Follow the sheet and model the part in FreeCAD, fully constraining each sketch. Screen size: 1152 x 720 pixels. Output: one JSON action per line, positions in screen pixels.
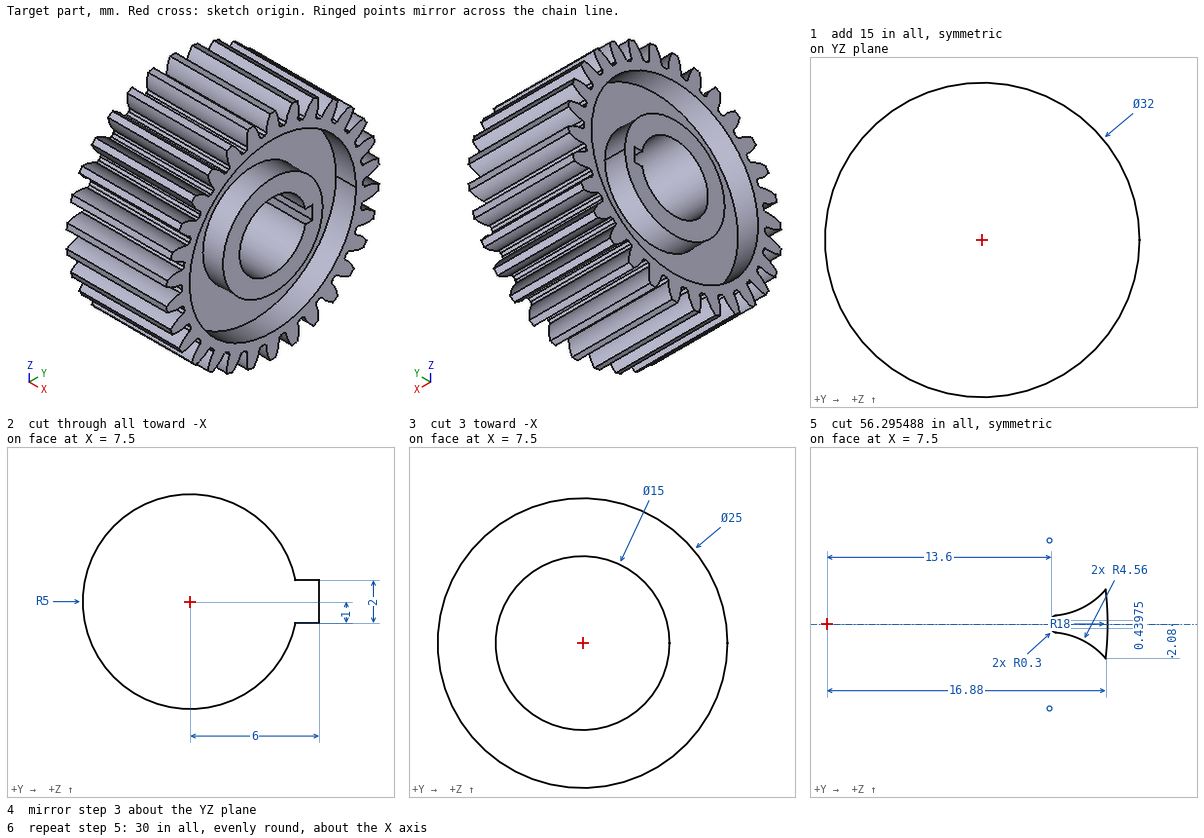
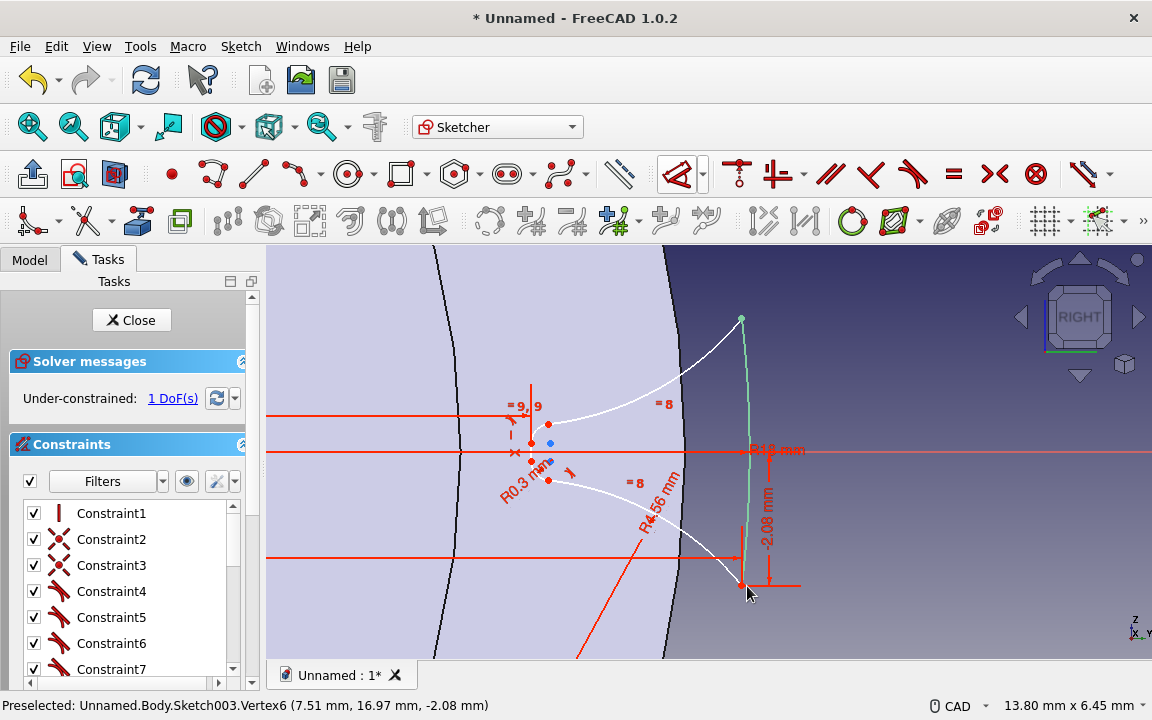
{"action": "scroll", "coordinate": [531, 452], "scroll_direction": "up", "scroll_amount": 3}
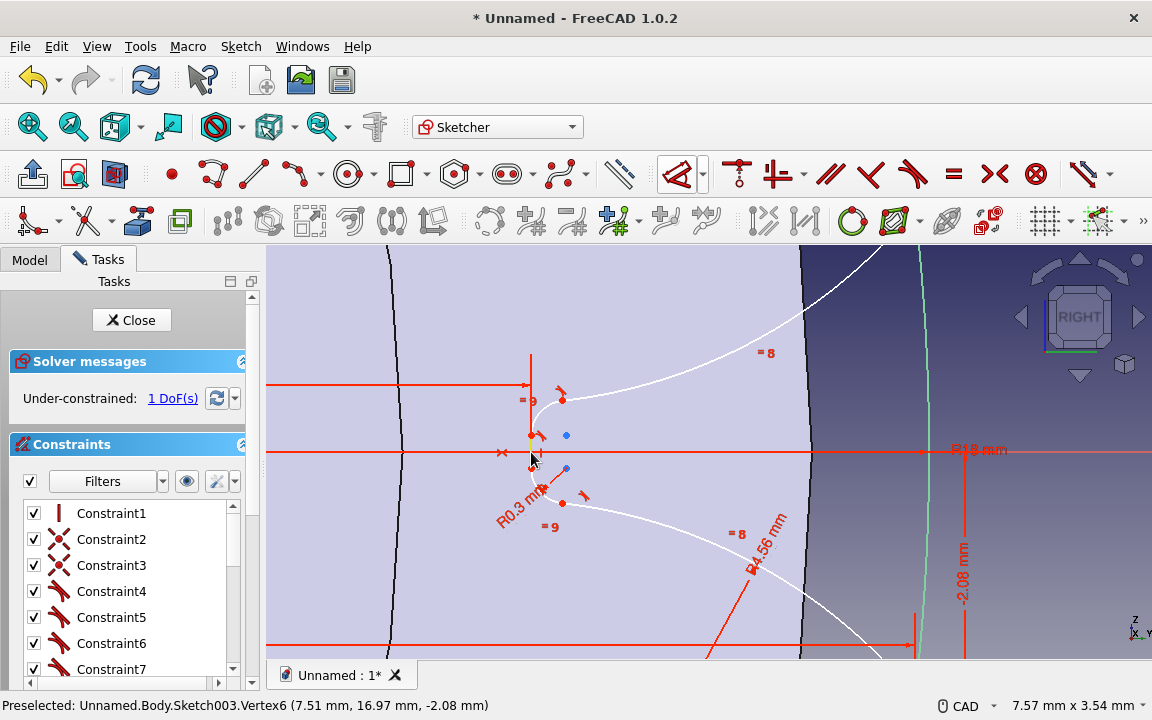
{"action": "left_click", "coordinate": [531, 452]}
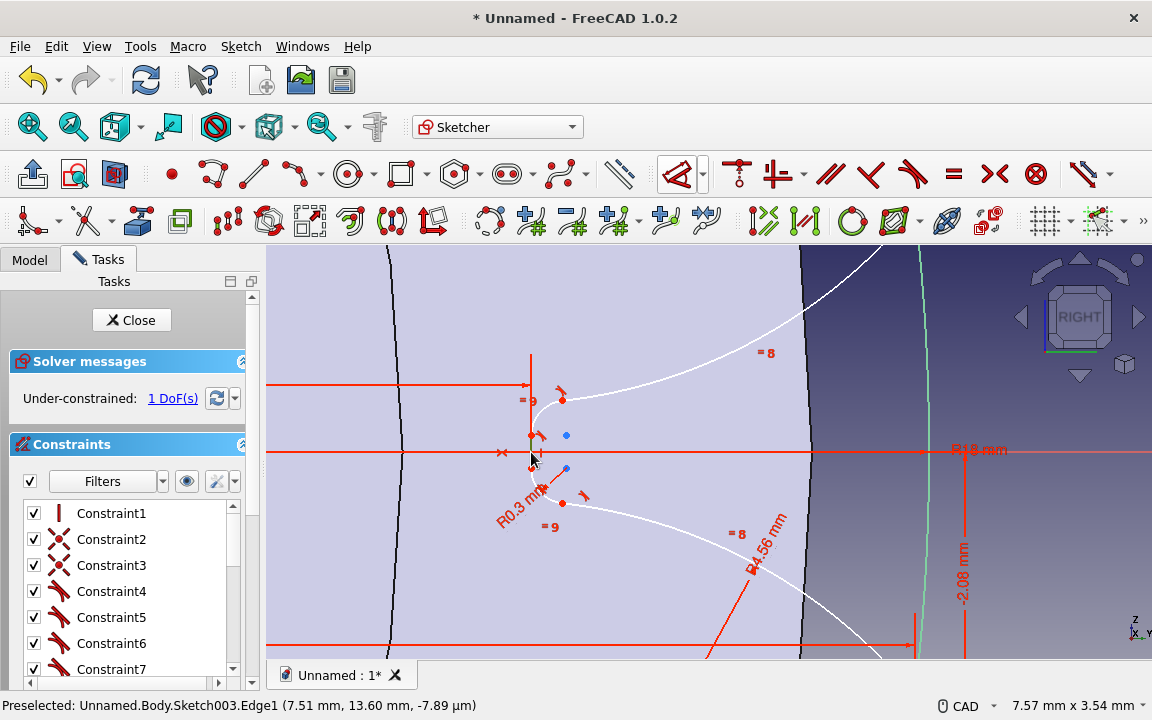
{"action": "key", "text": "i"}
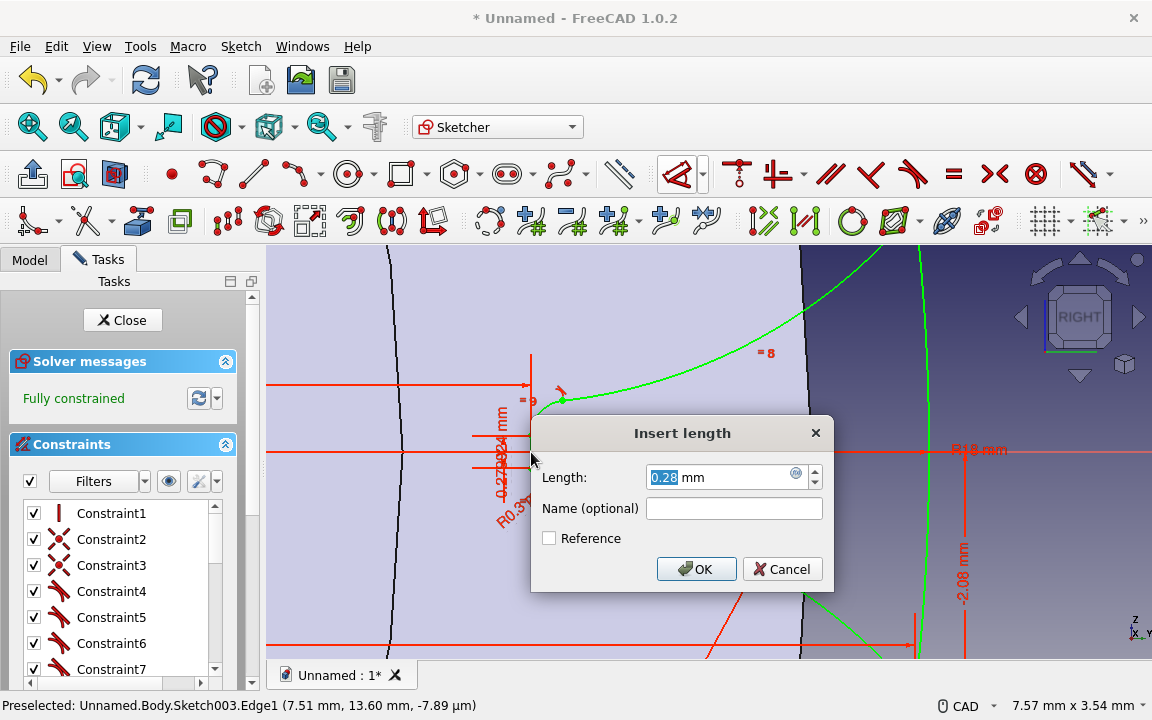
{"action": "type", "text": "0.43975"}
{"action": "key", "text": "Return"}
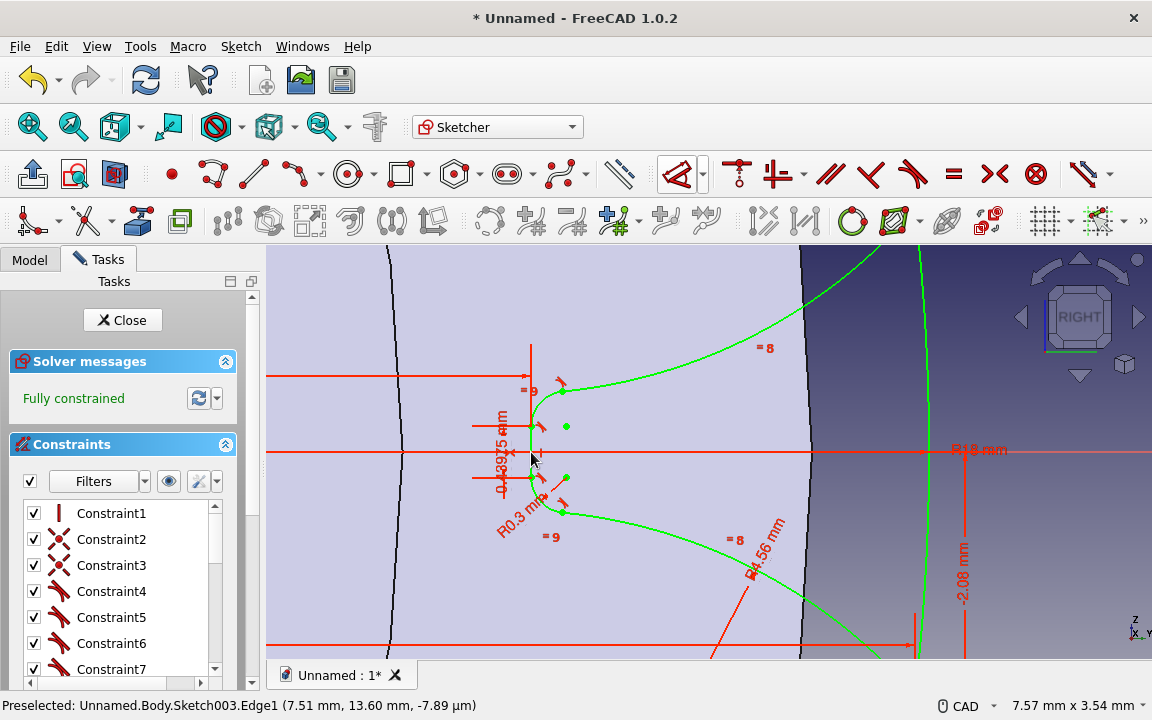
{"action": "left_click", "coordinate": [123, 320]}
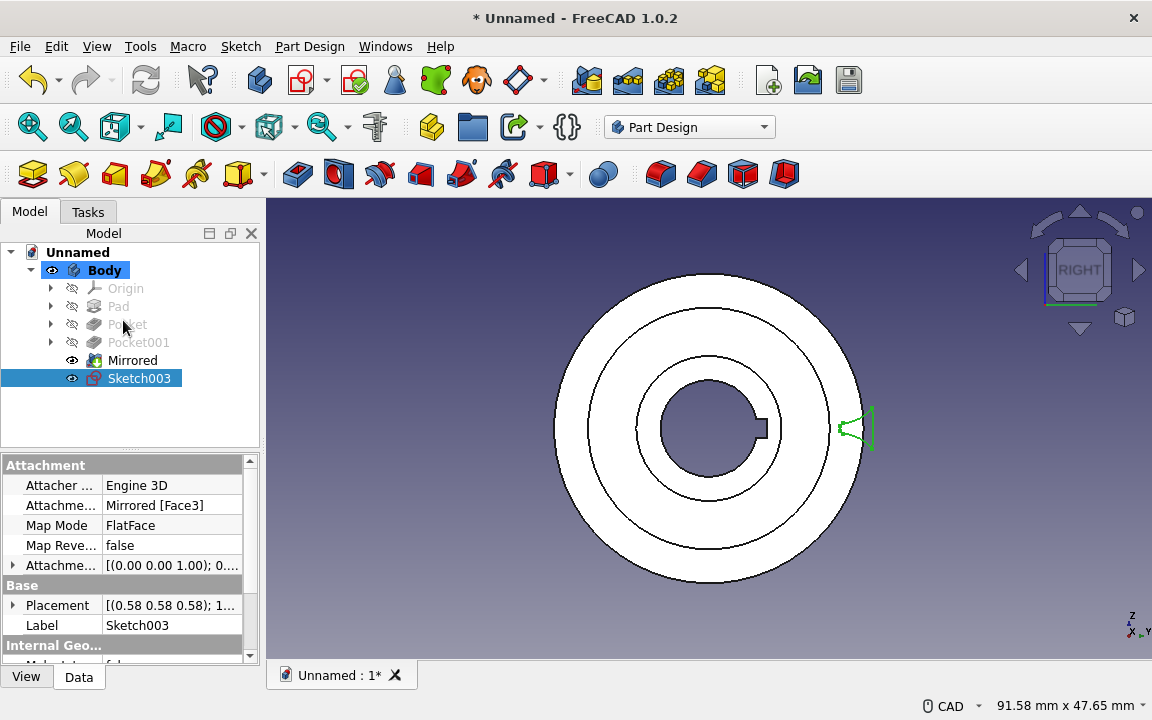
{"action": "left_click", "coordinate": [298, 174]}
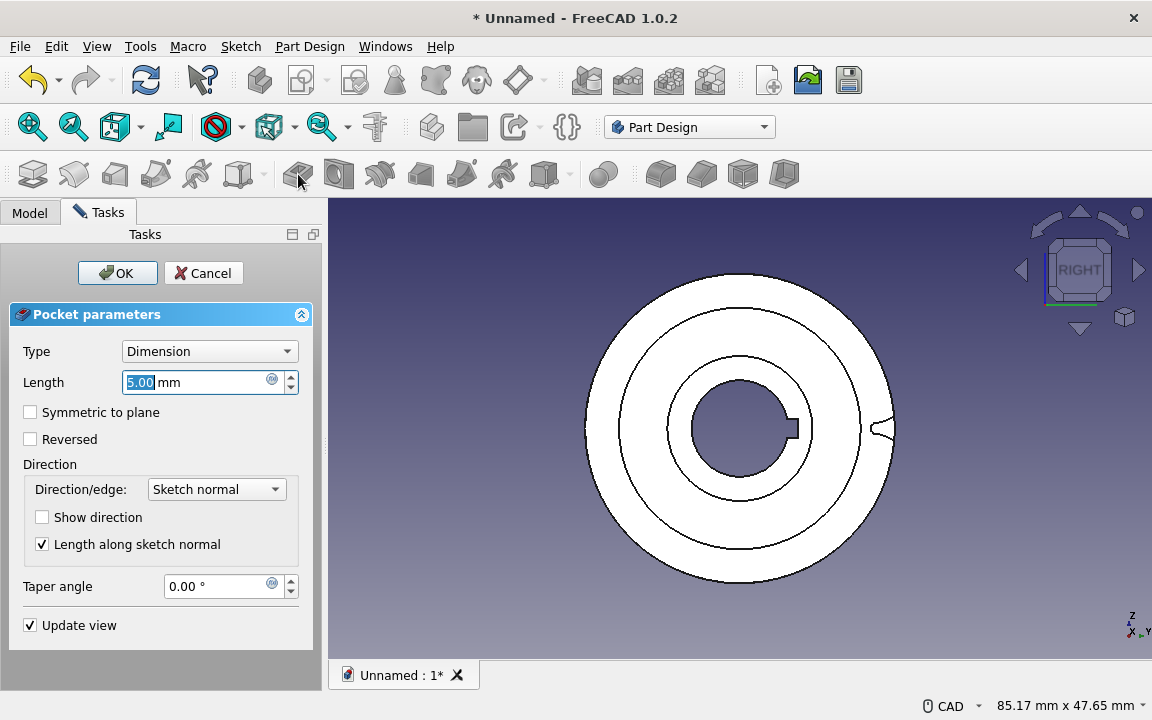
{"action": "type", "text": "56.295488"}
{"action": "key", "text": "Tab"}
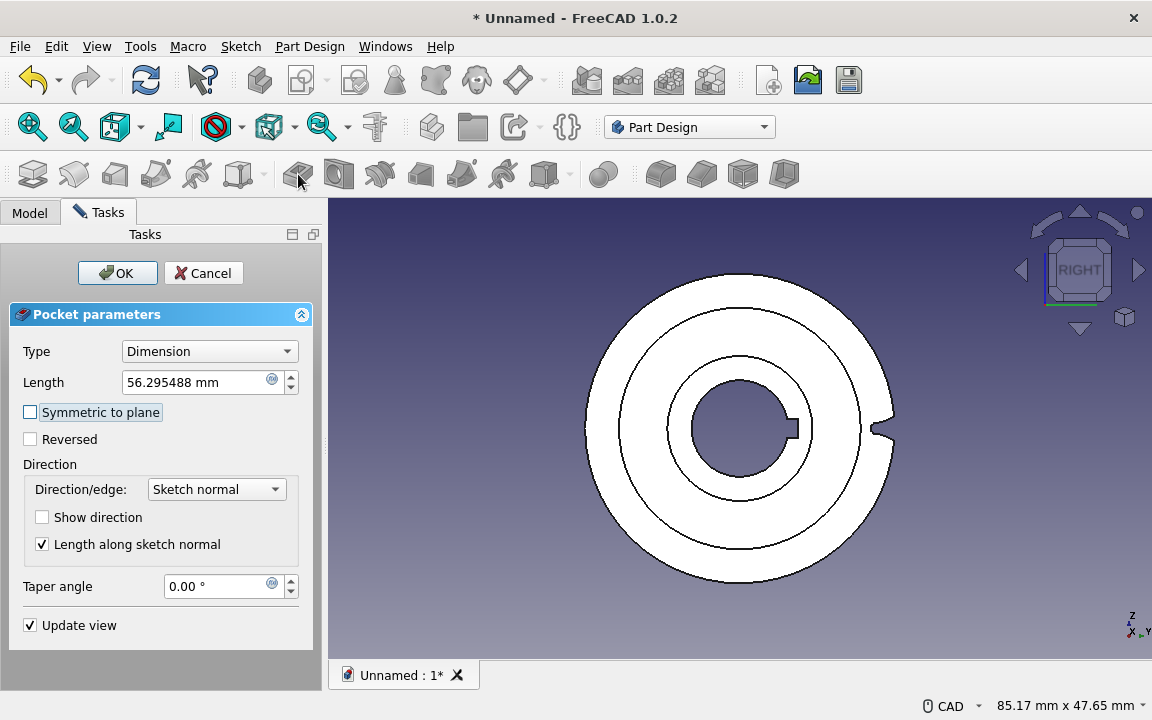
{"action": "left_click", "coordinate": [31, 412]}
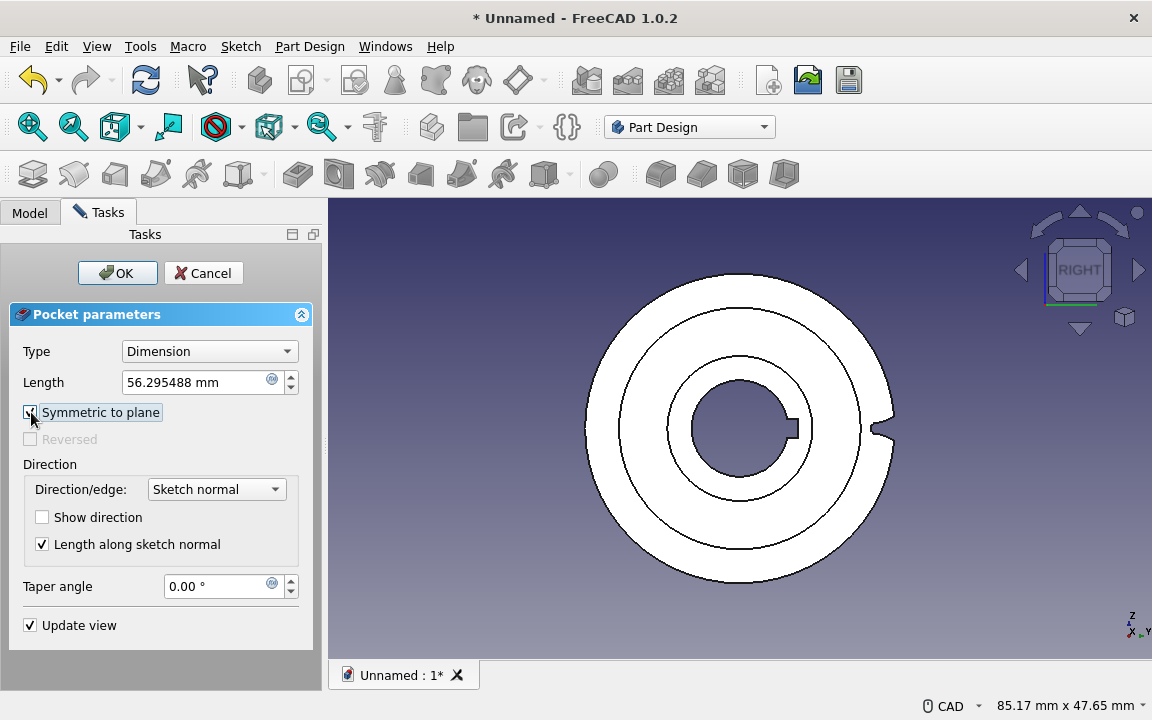
{"action": "left_click", "coordinate": [118, 273]}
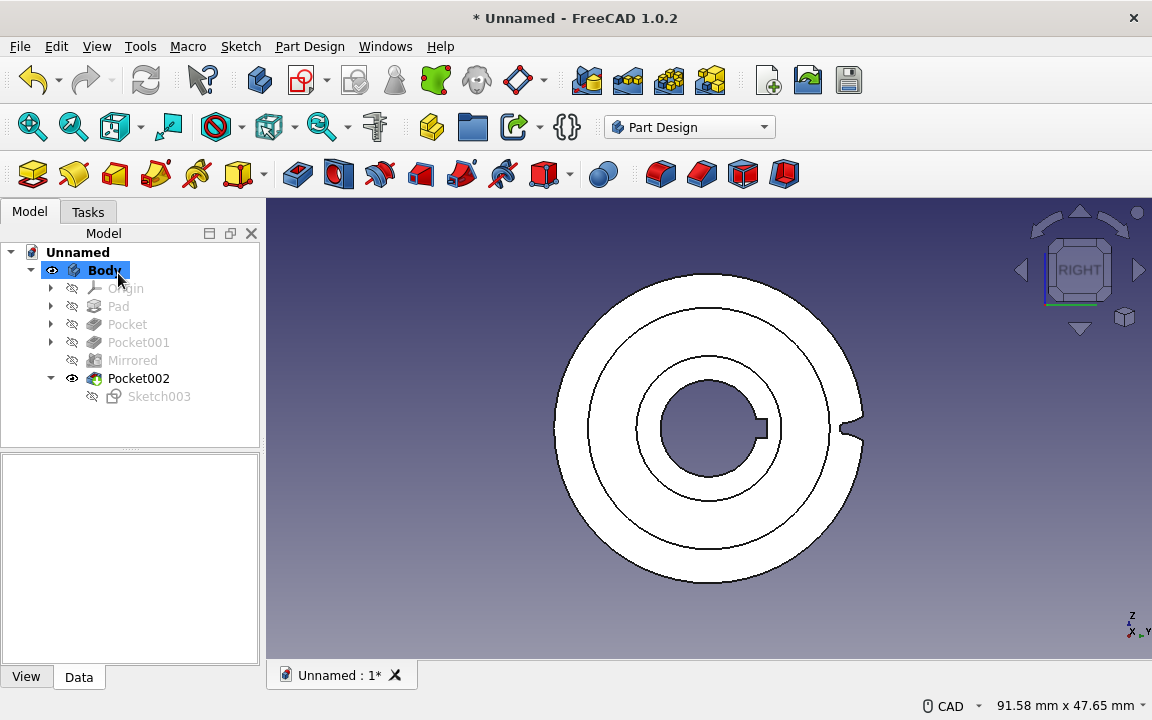
{"action": "left_click", "coordinate": [117, 378]}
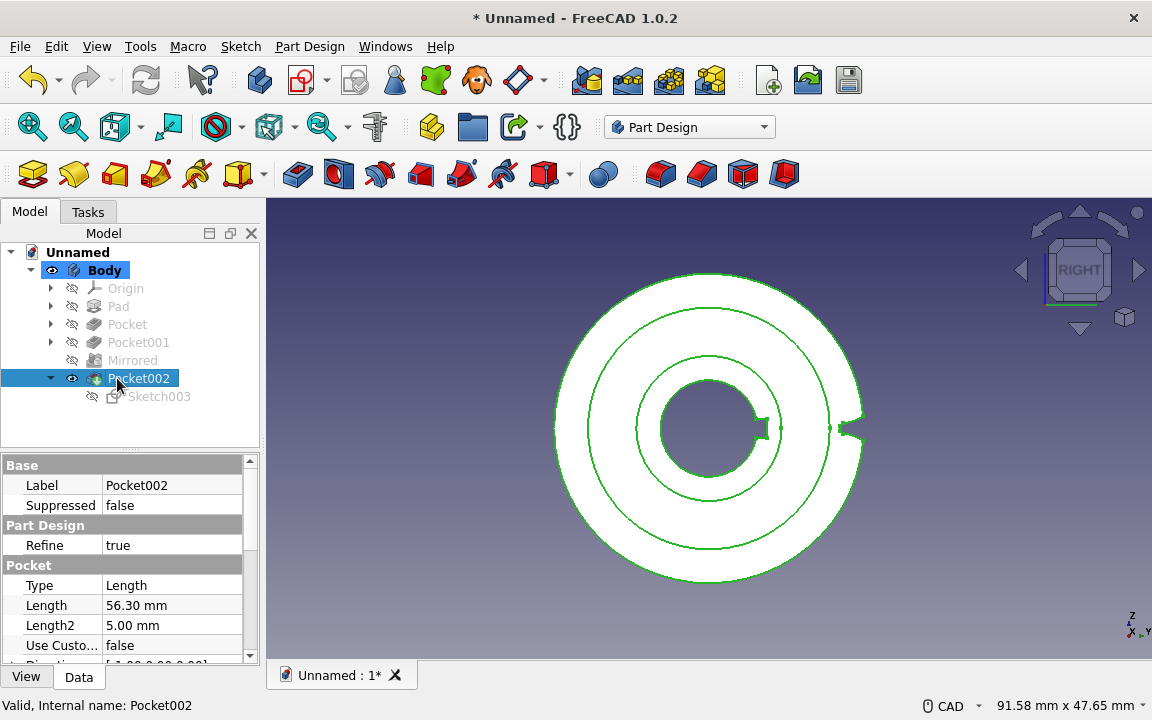
{"action": "left_click", "coordinate": [669, 80]}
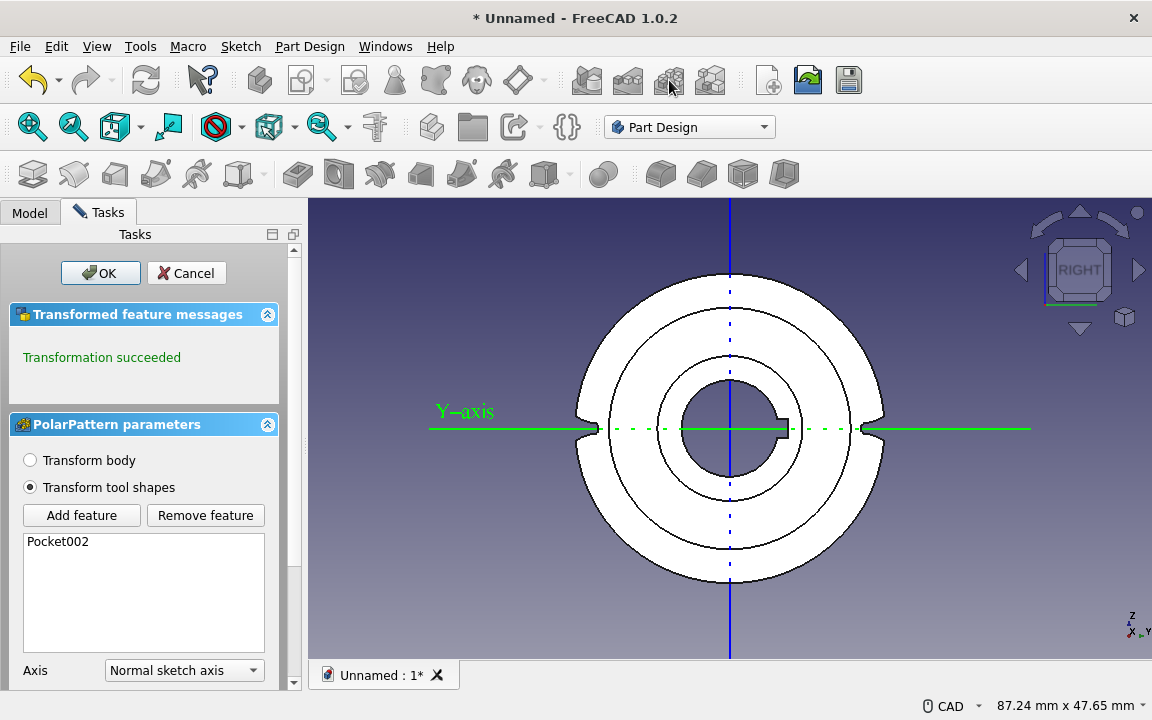
{"action": "left_click", "coordinate": [185, 670]}